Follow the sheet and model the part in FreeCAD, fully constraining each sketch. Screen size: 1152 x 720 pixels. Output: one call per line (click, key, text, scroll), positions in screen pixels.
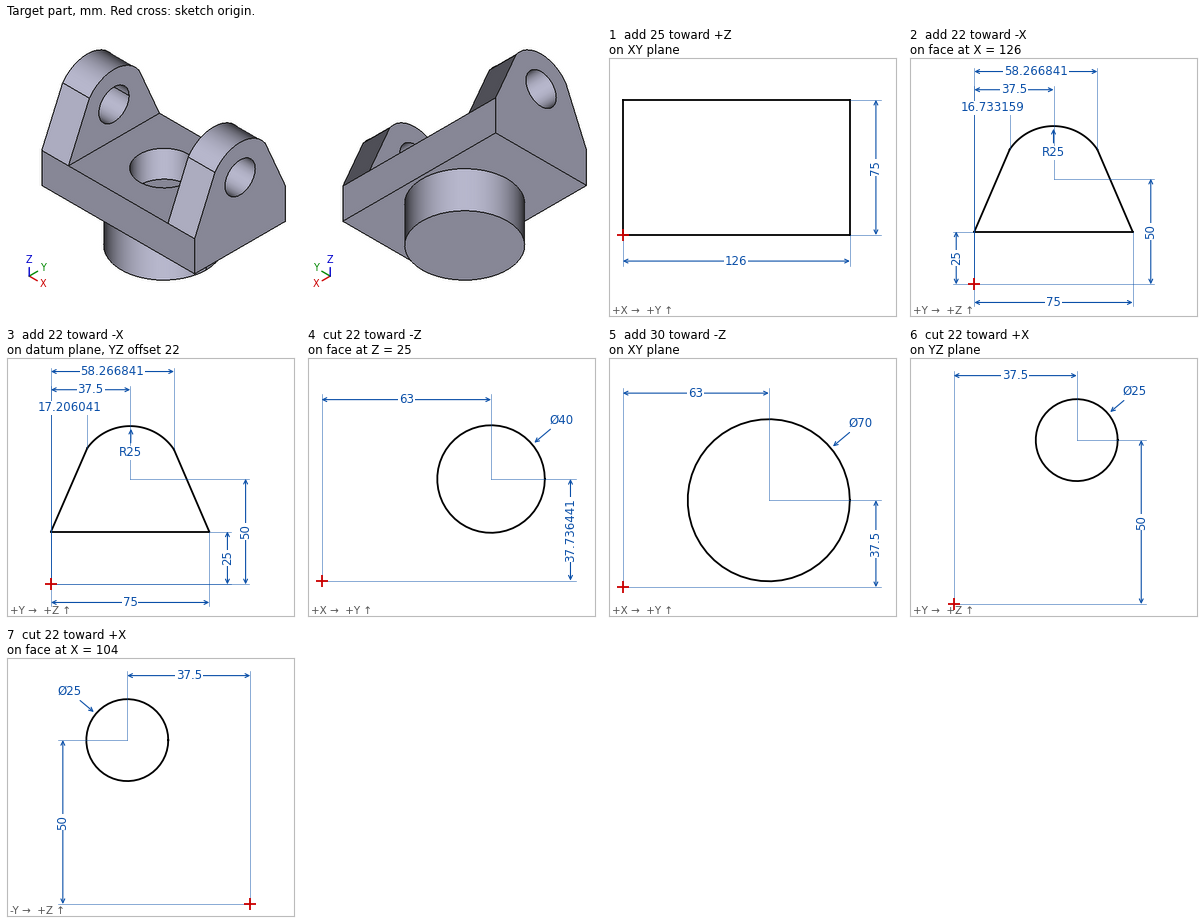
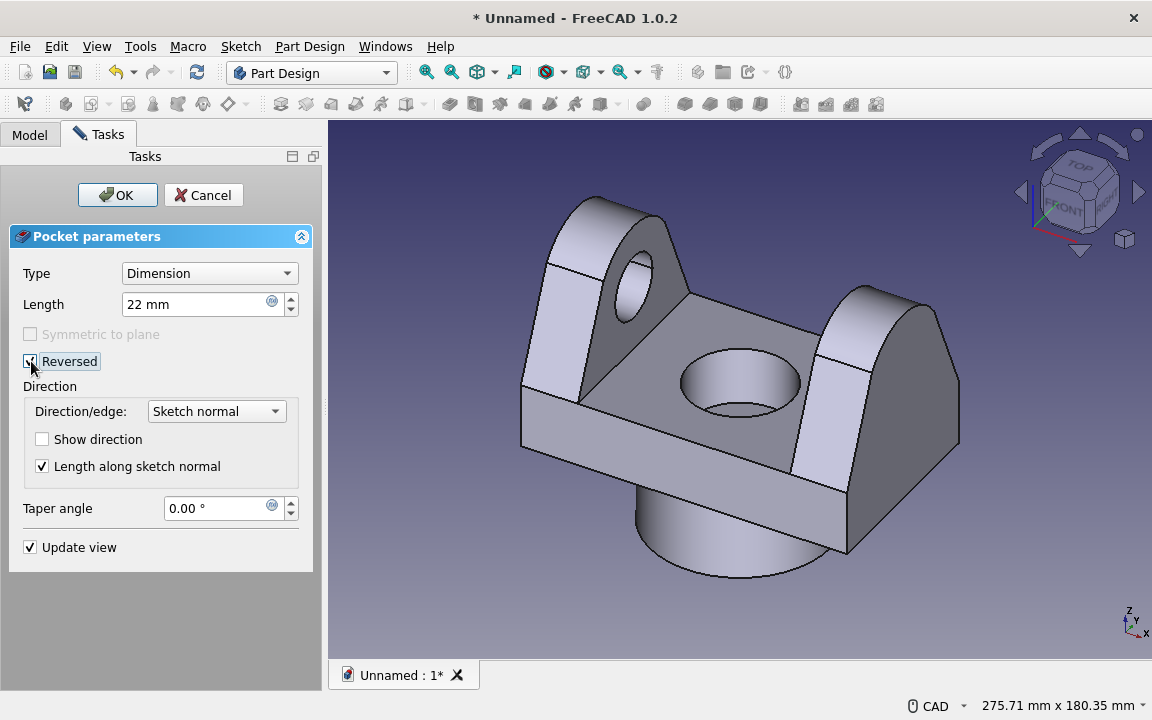
click(118, 195)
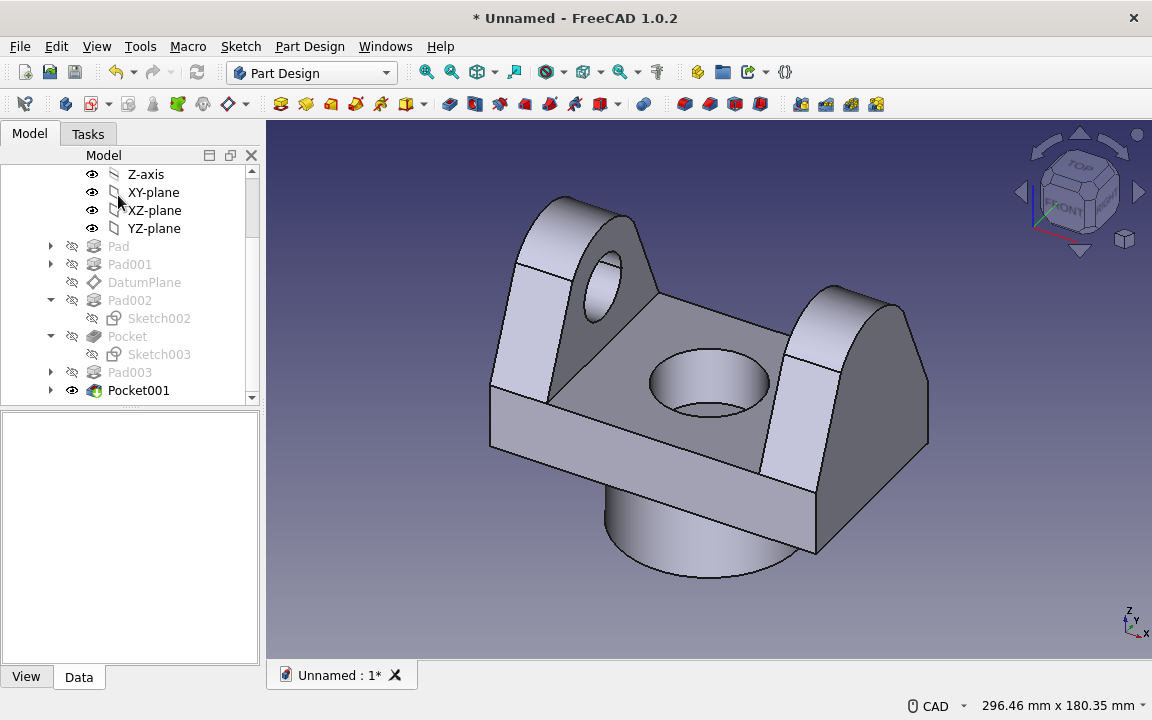
key(6)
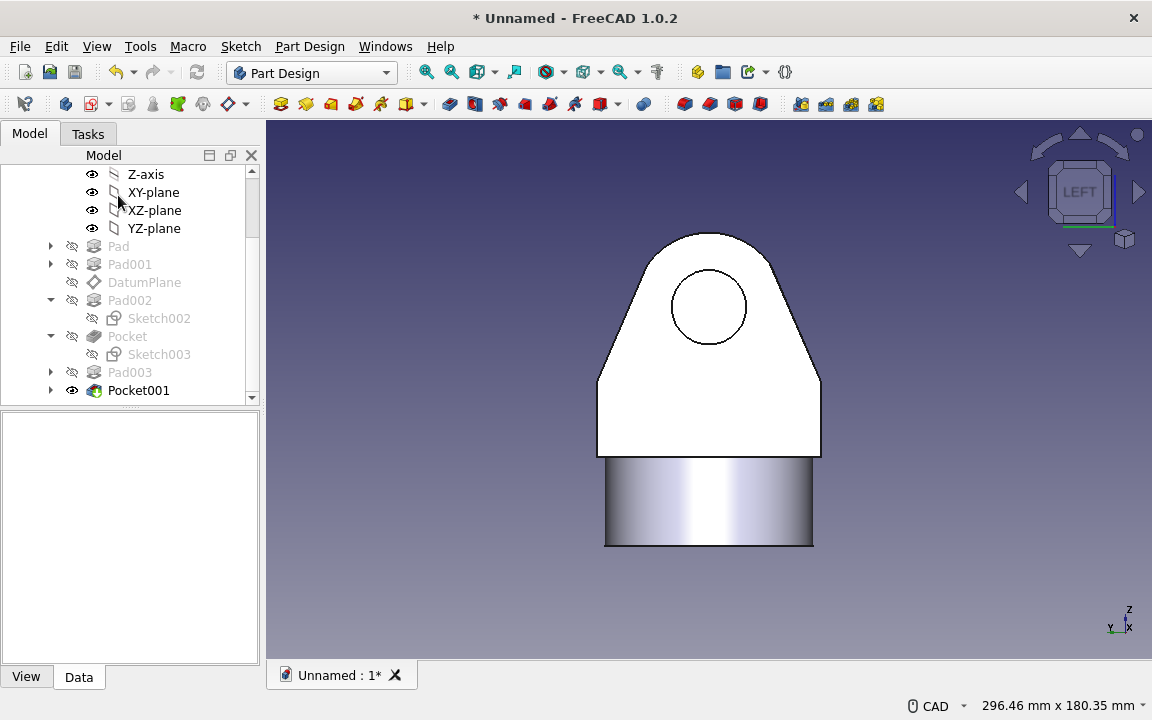
click(709, 306)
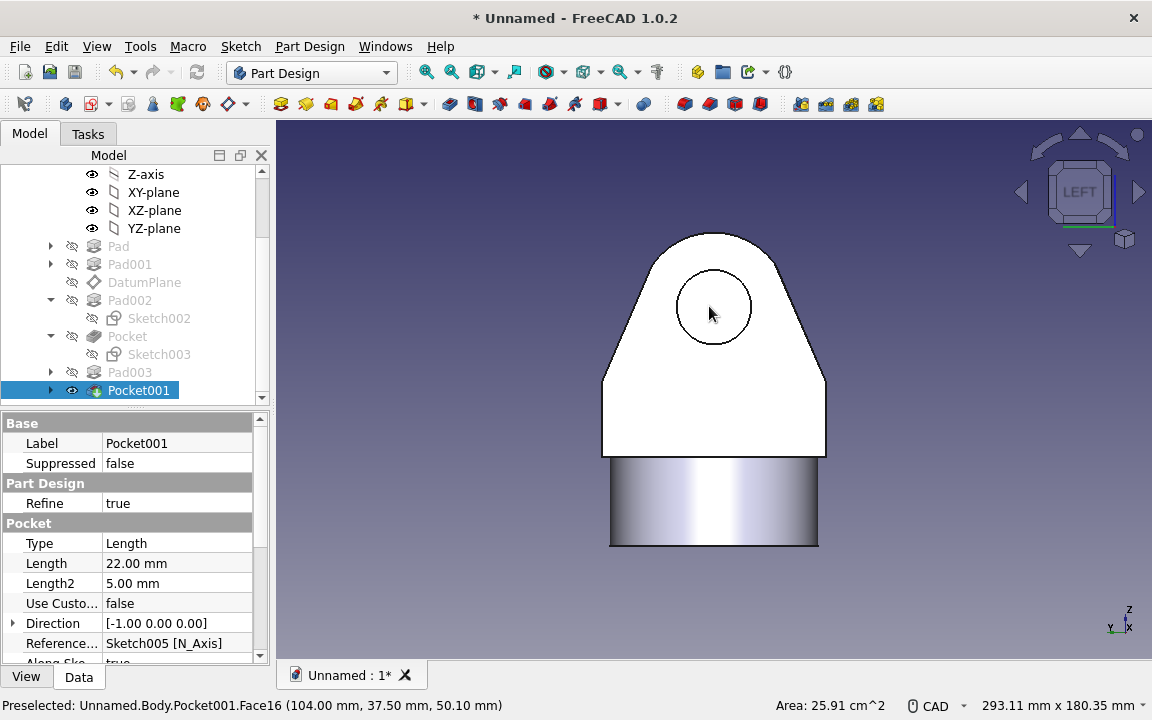
click(90, 104)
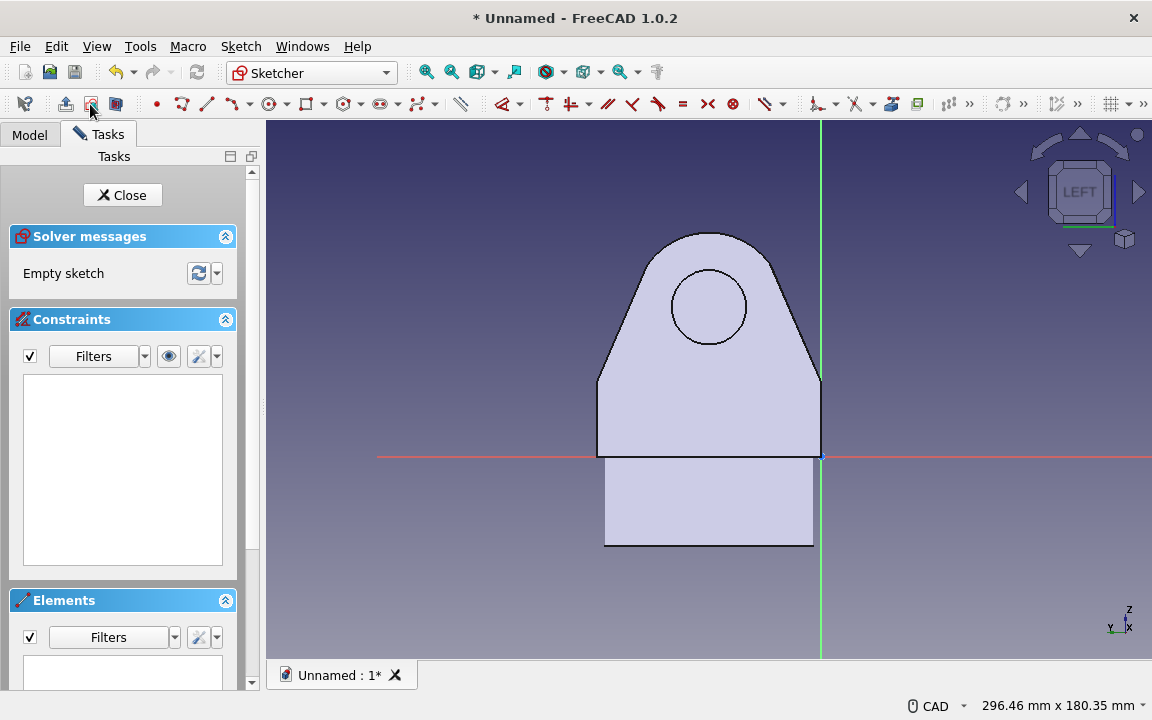
click(116, 104)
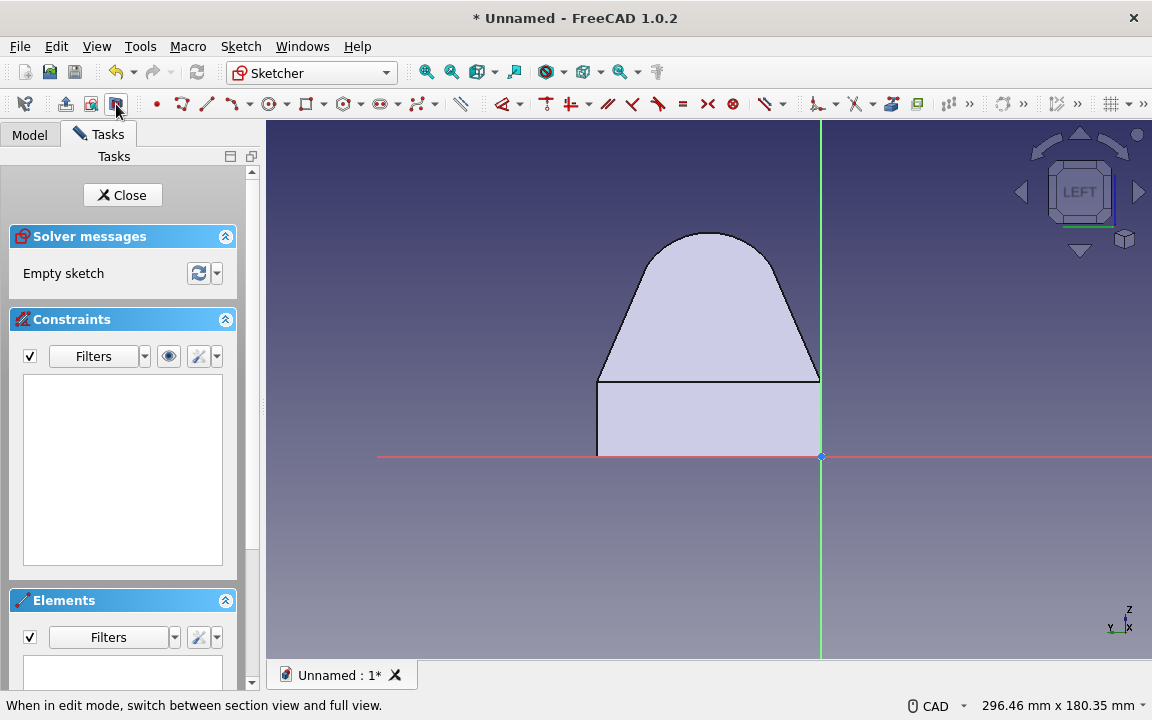
scroll(726, 287, up, 8)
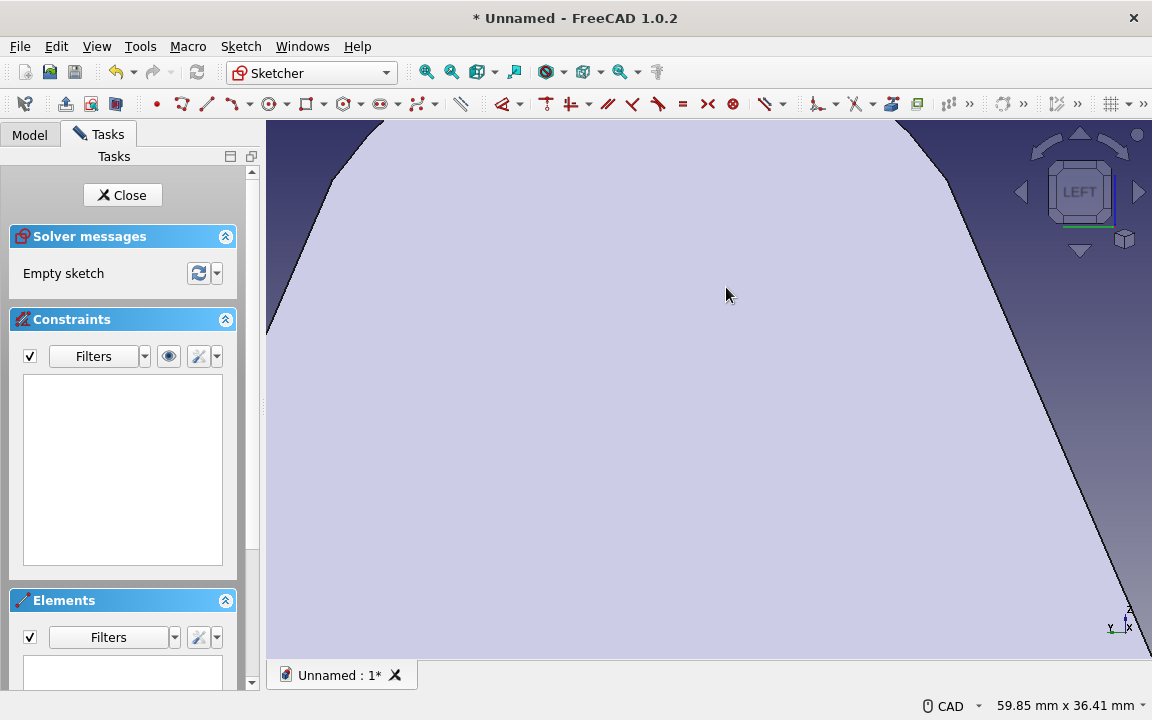
click(268, 104)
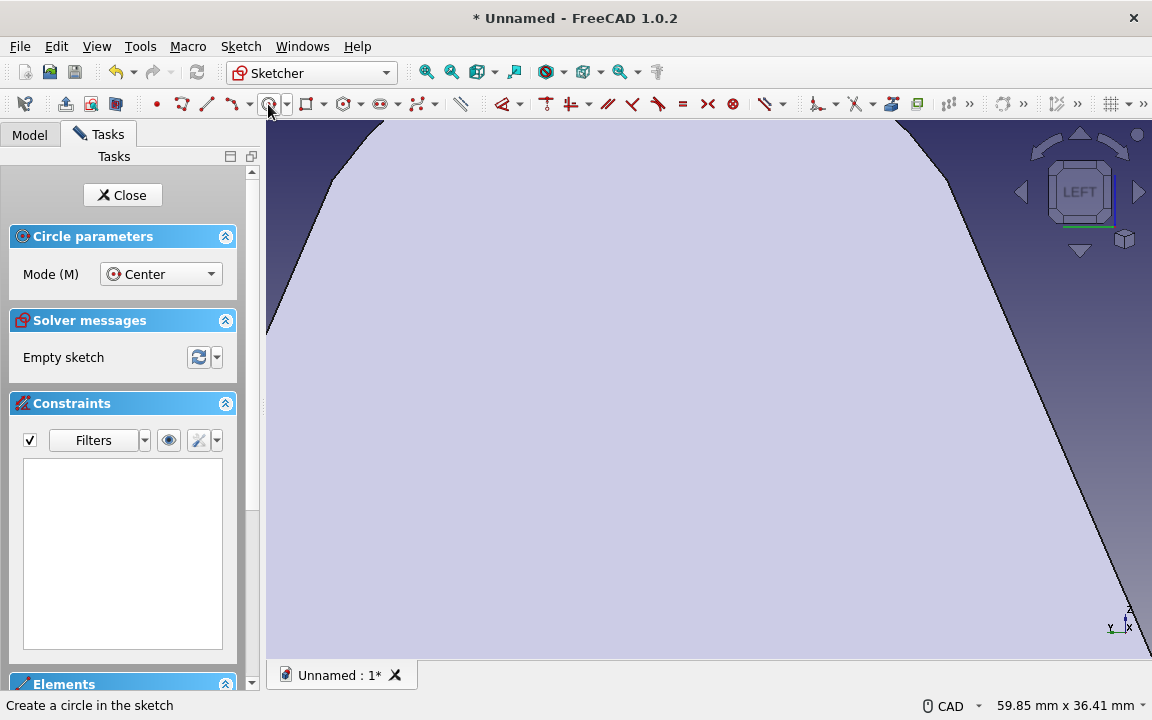
click(640, 386)
move(771, 256)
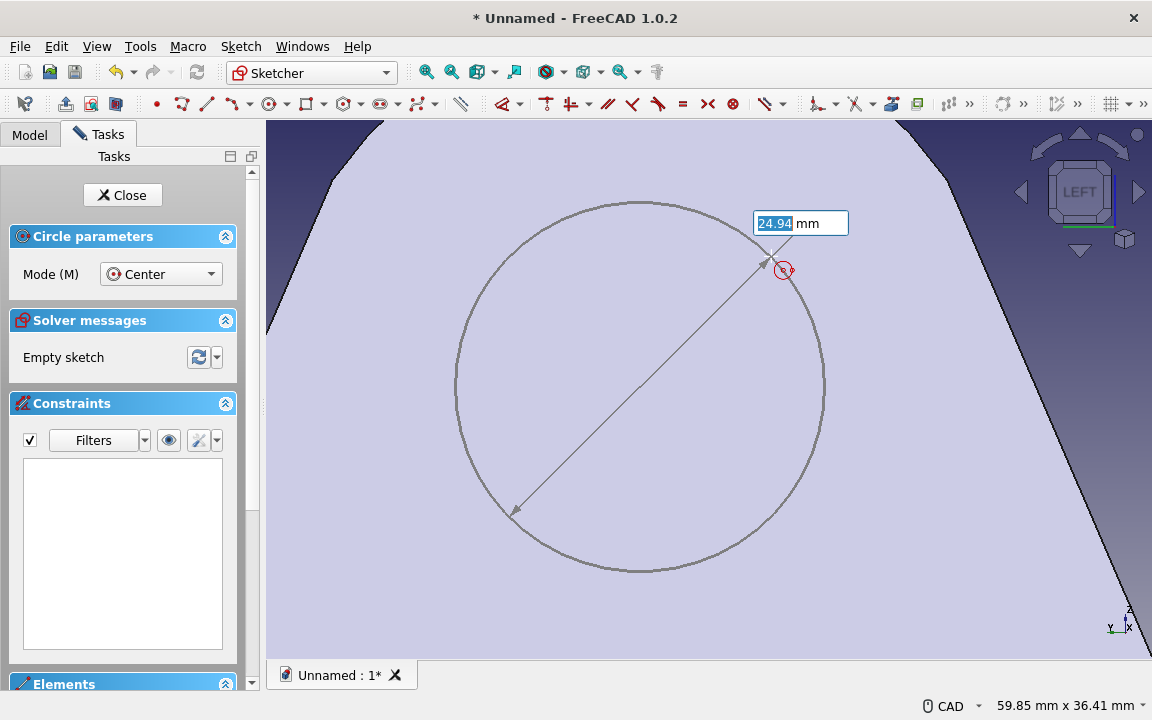
text(25)
key(Return)
key(Escape)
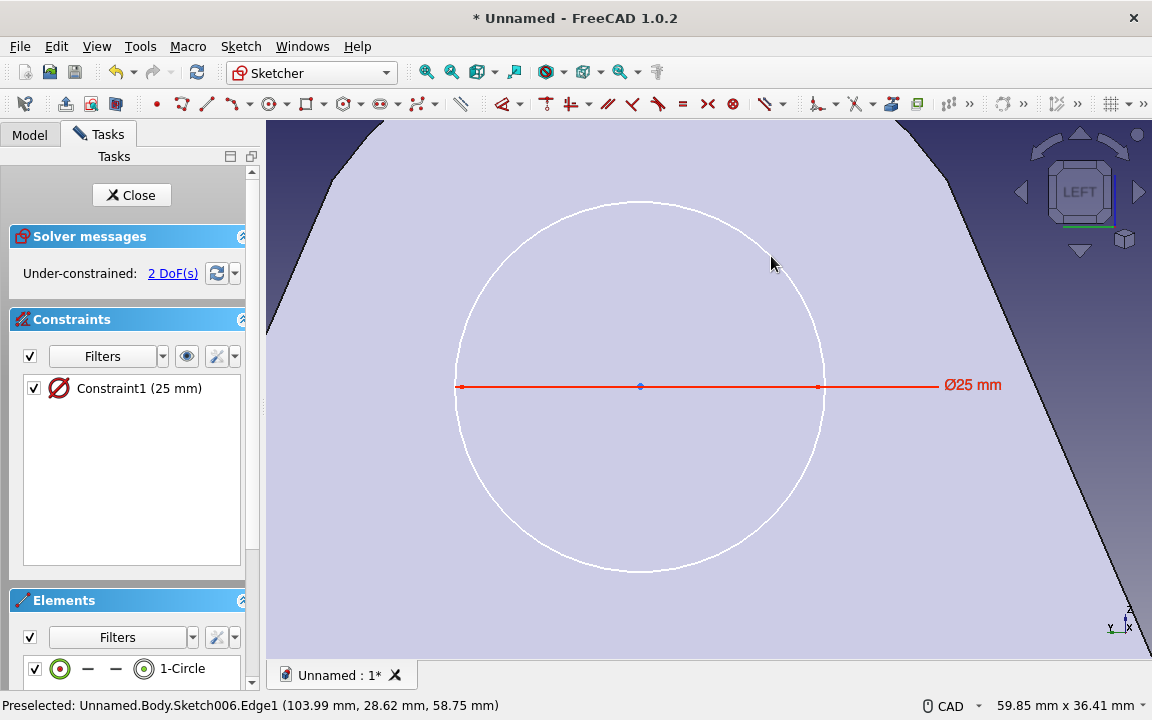
click(502, 104)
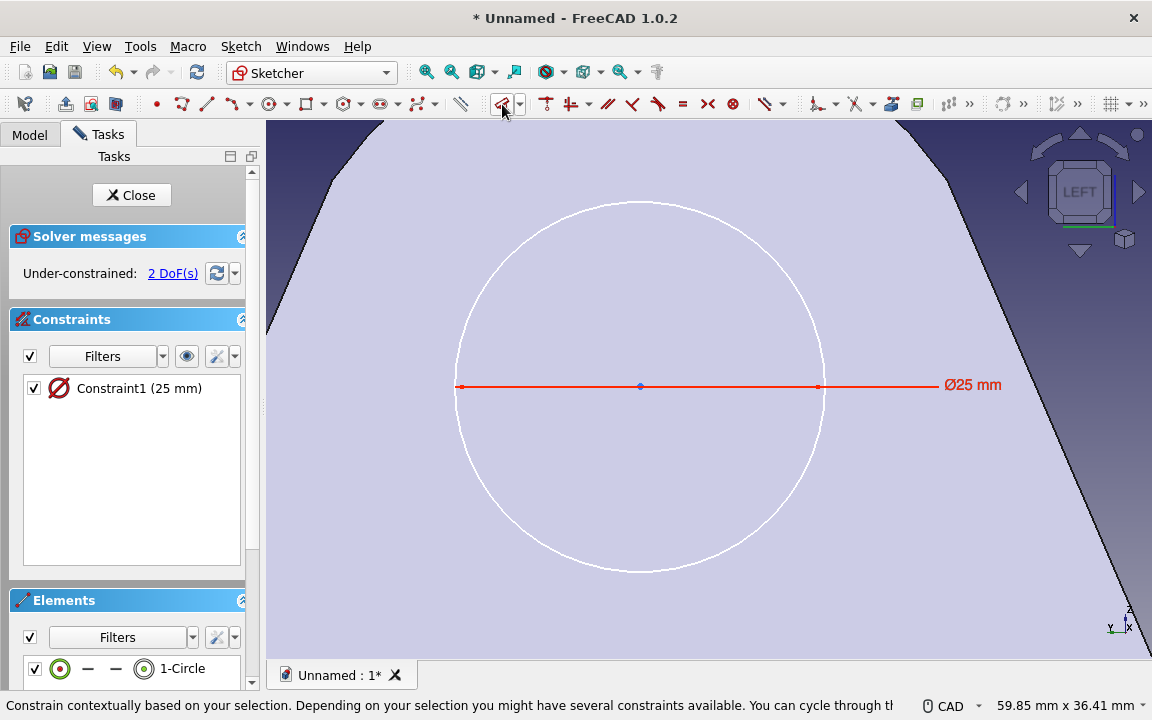
click(640, 387)
click(606, 509)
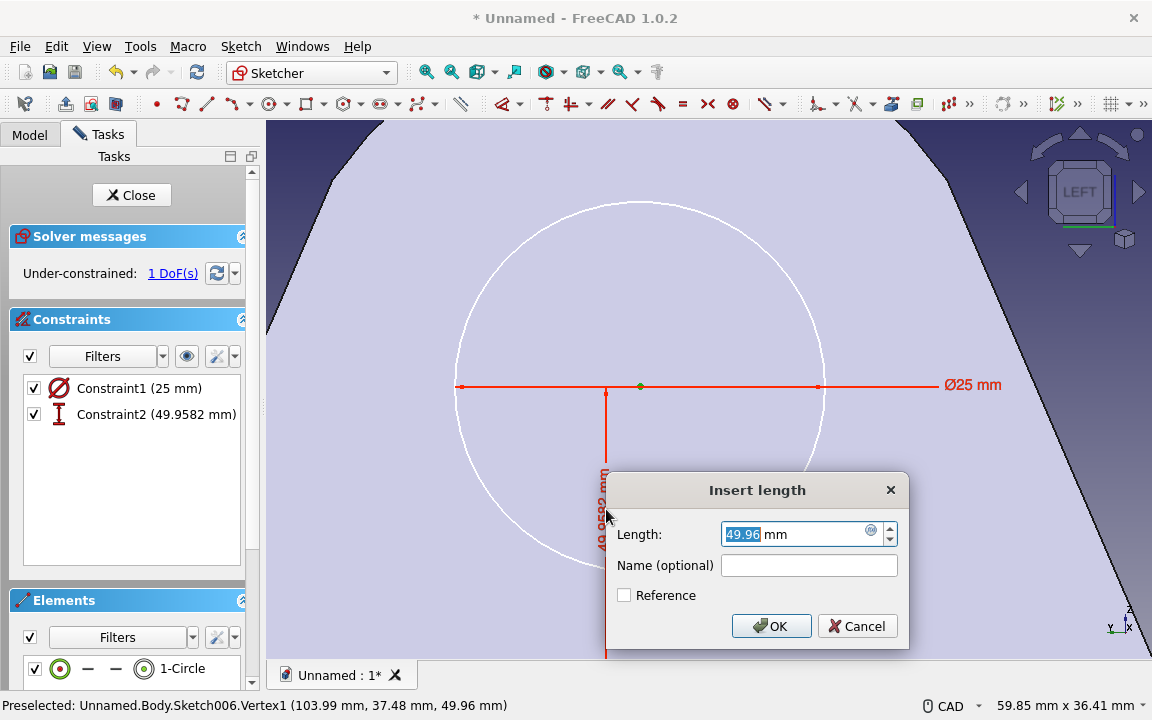
text(50)
key(Return)